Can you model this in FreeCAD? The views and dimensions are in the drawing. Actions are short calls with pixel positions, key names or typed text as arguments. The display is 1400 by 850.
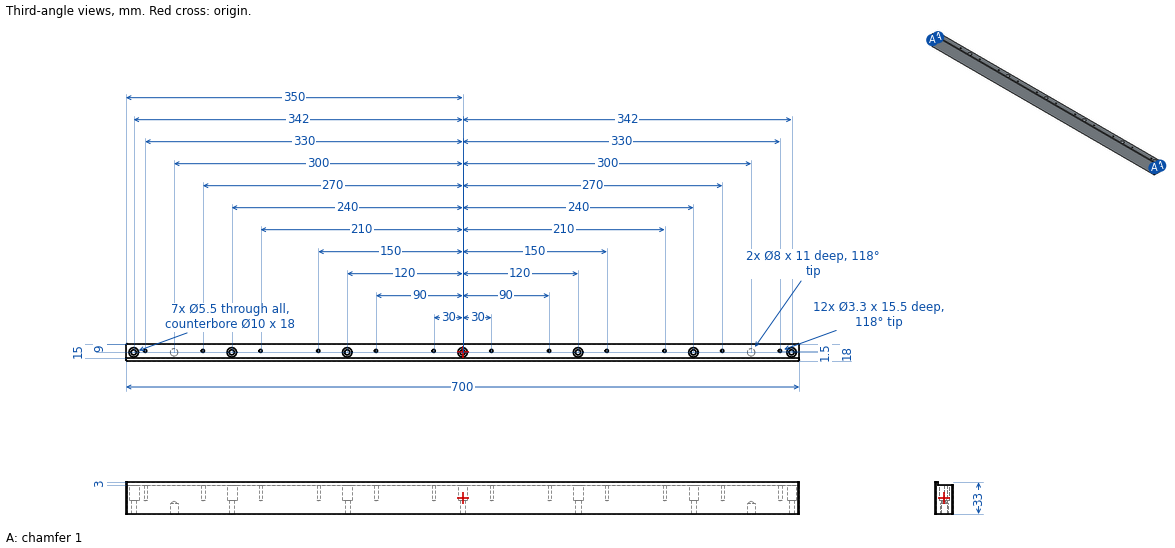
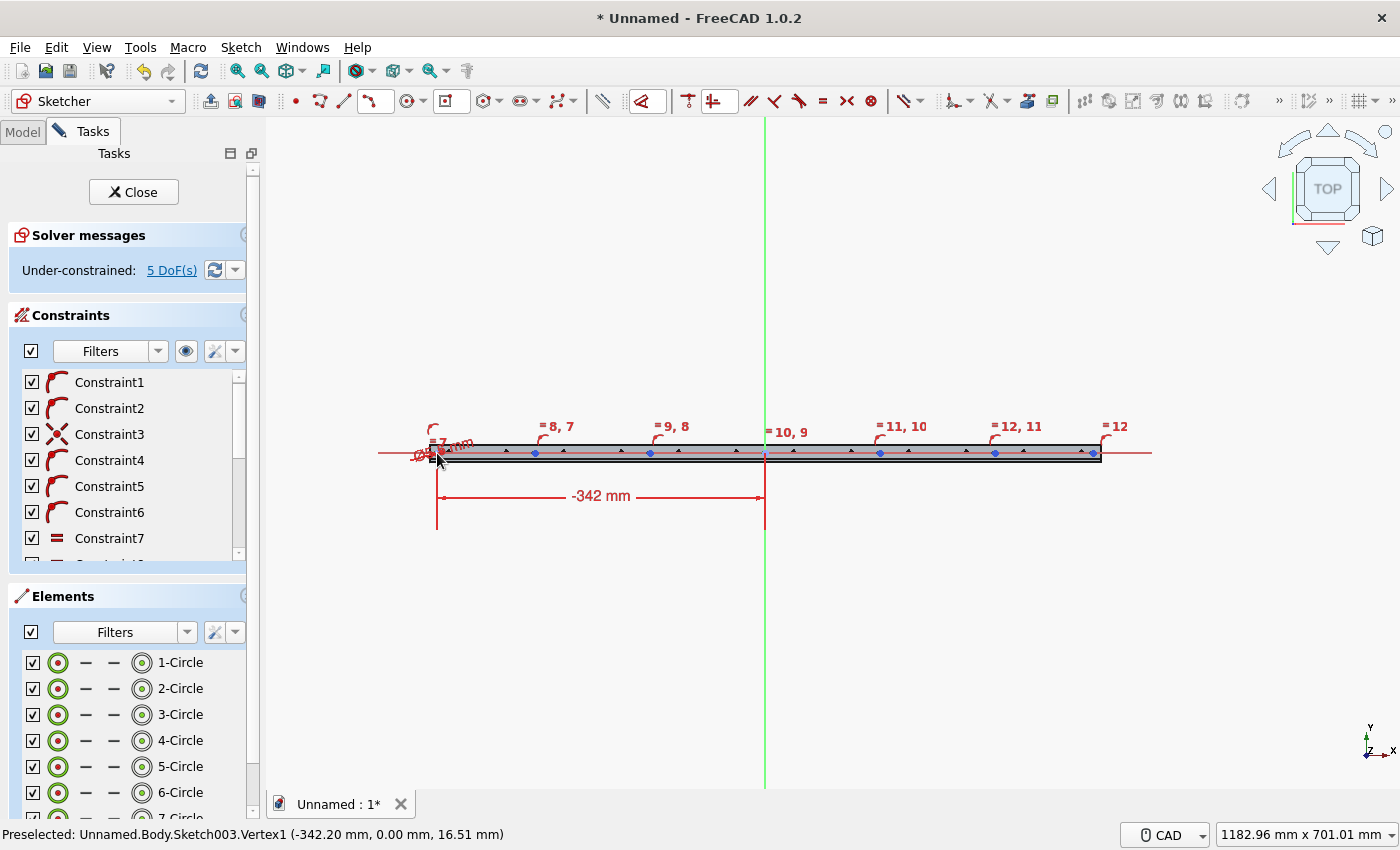
click(535, 453)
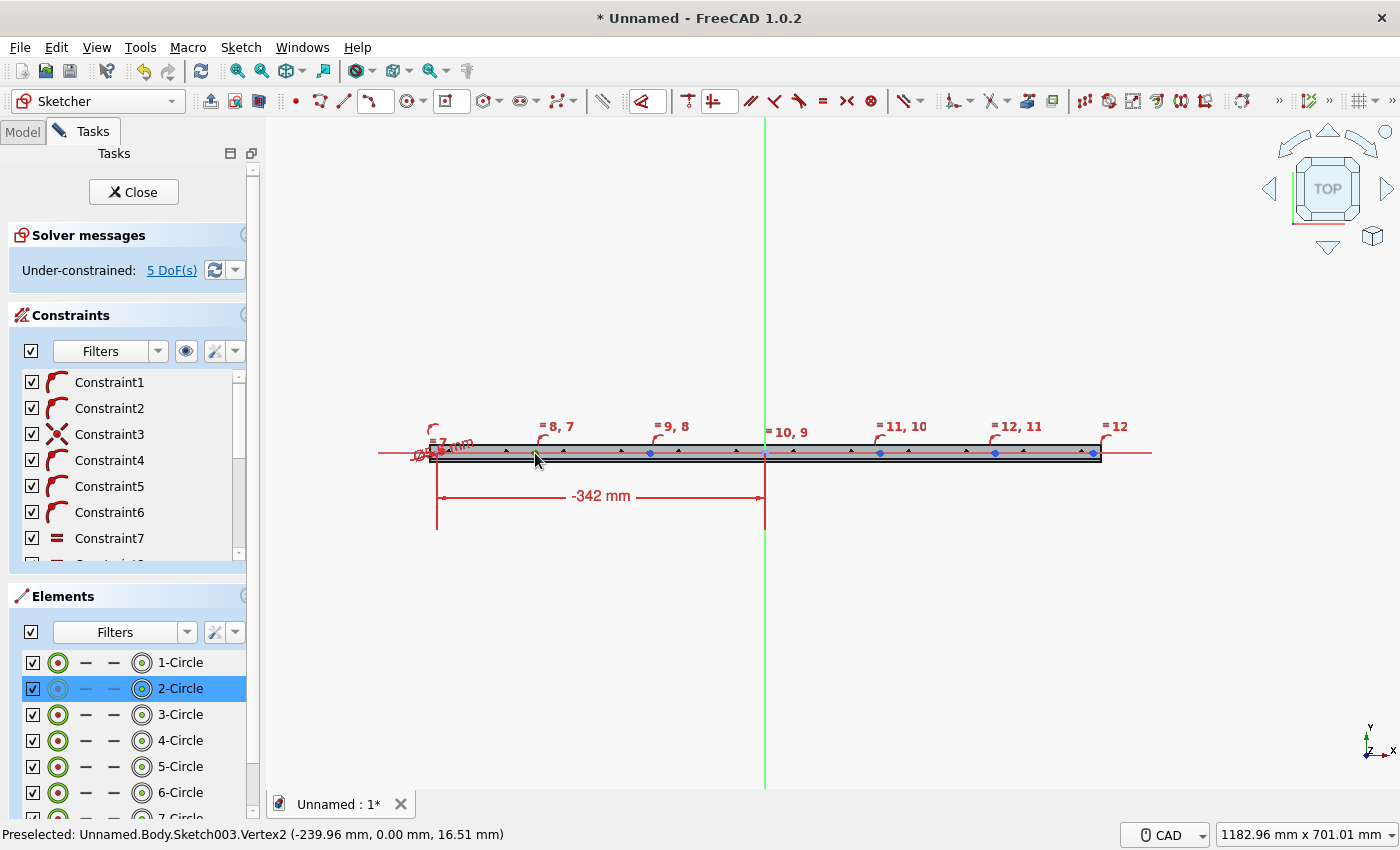
click(660, 102)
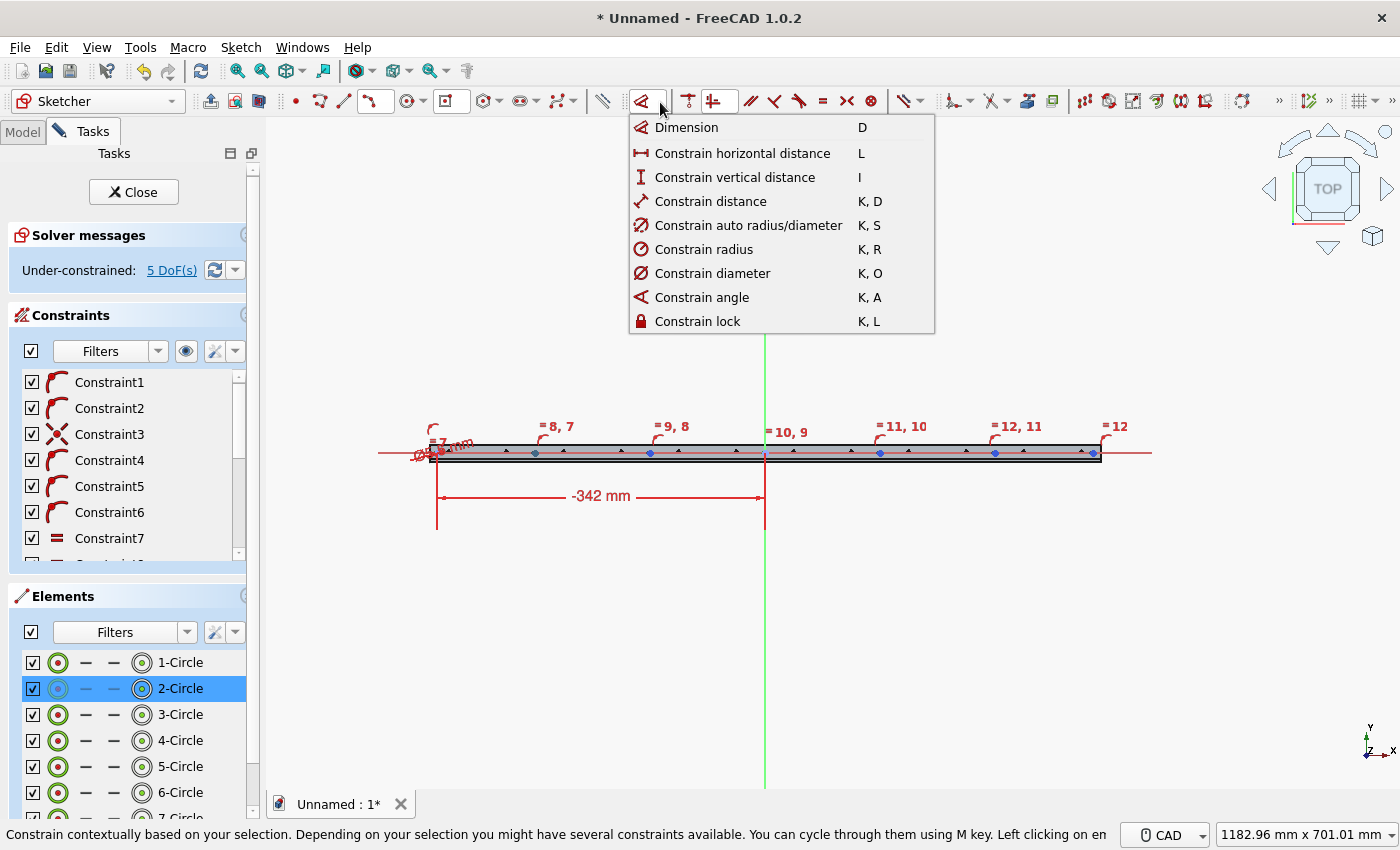
click(782, 153)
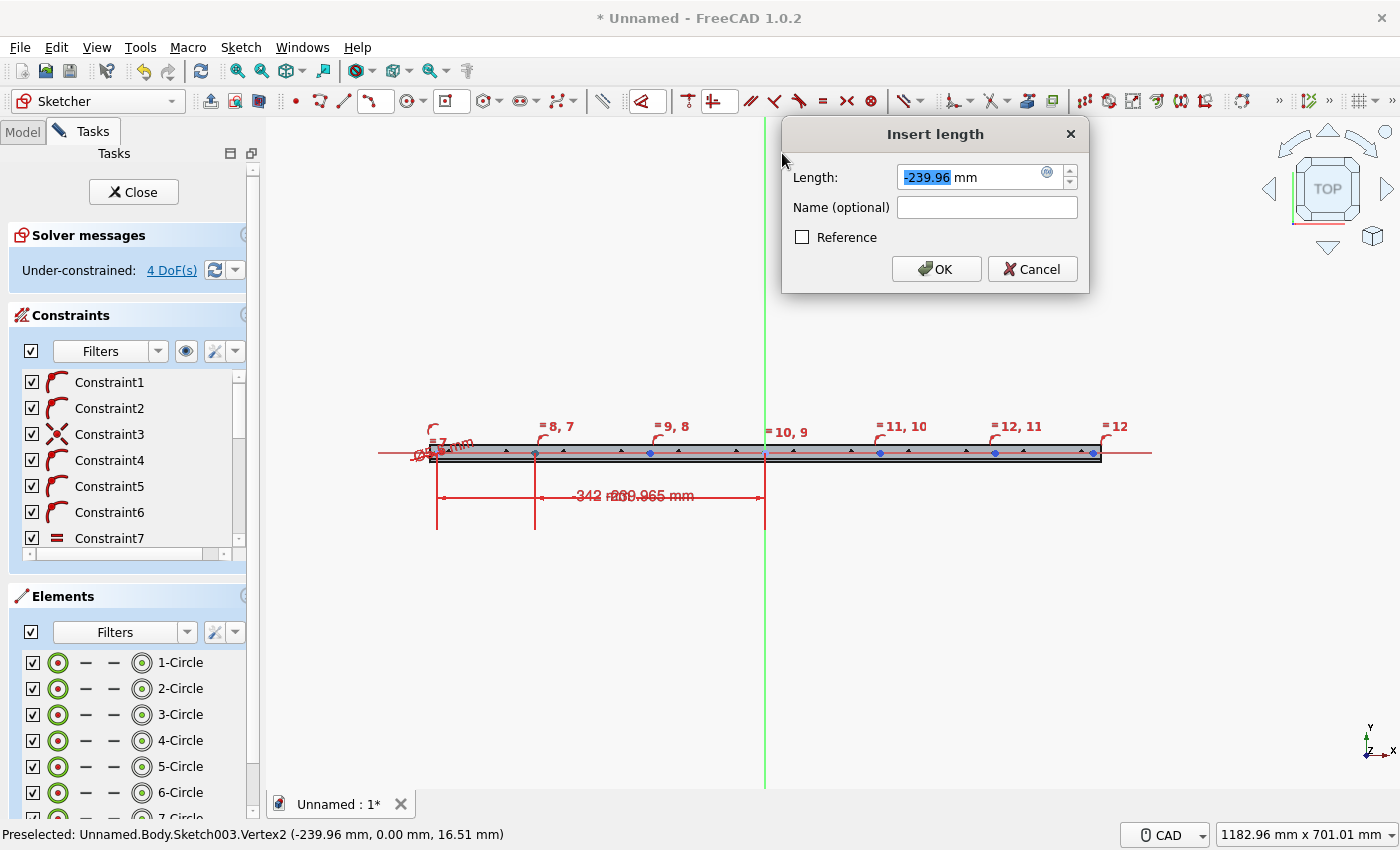
text(-240)
key(Return)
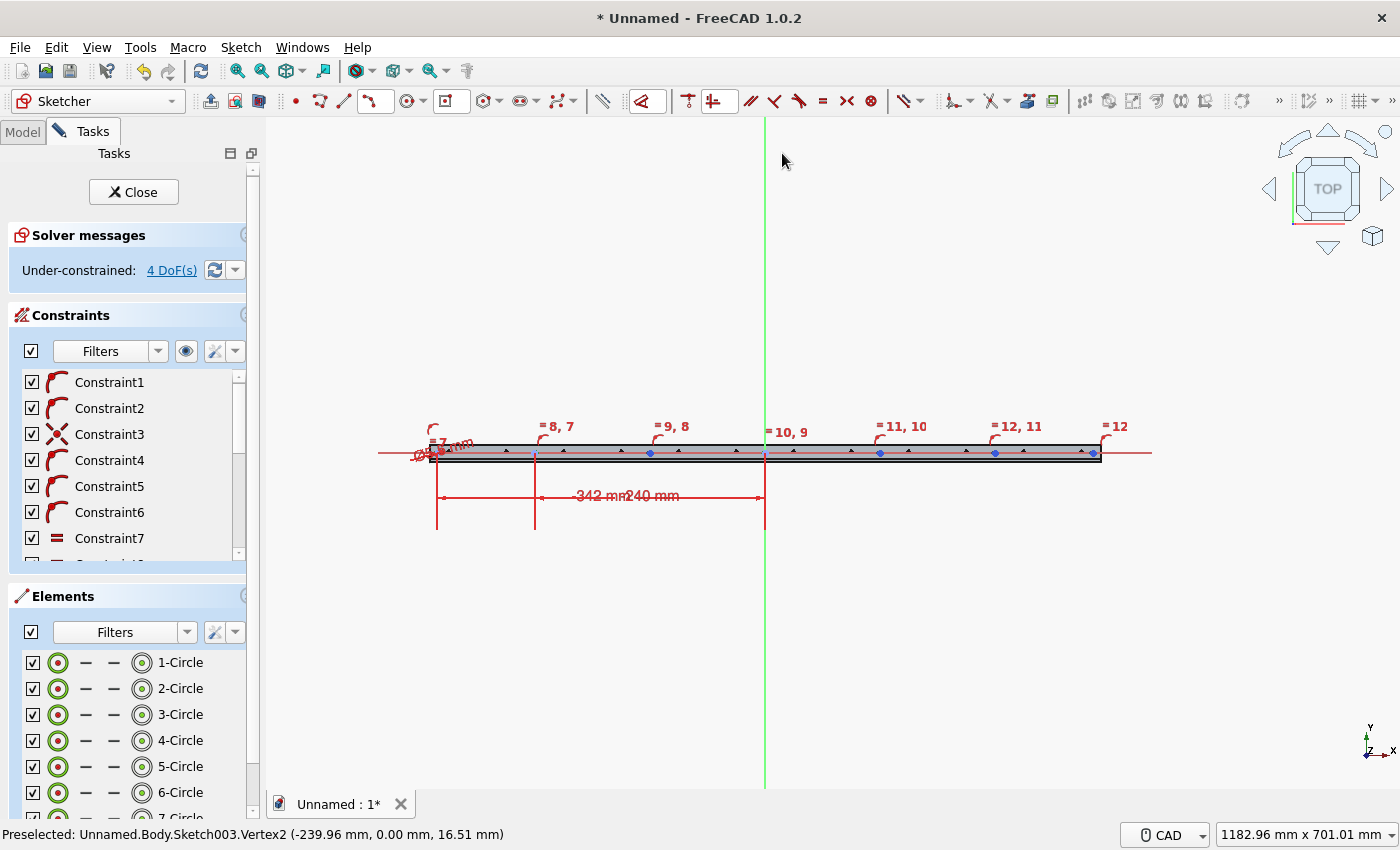
click(650, 453)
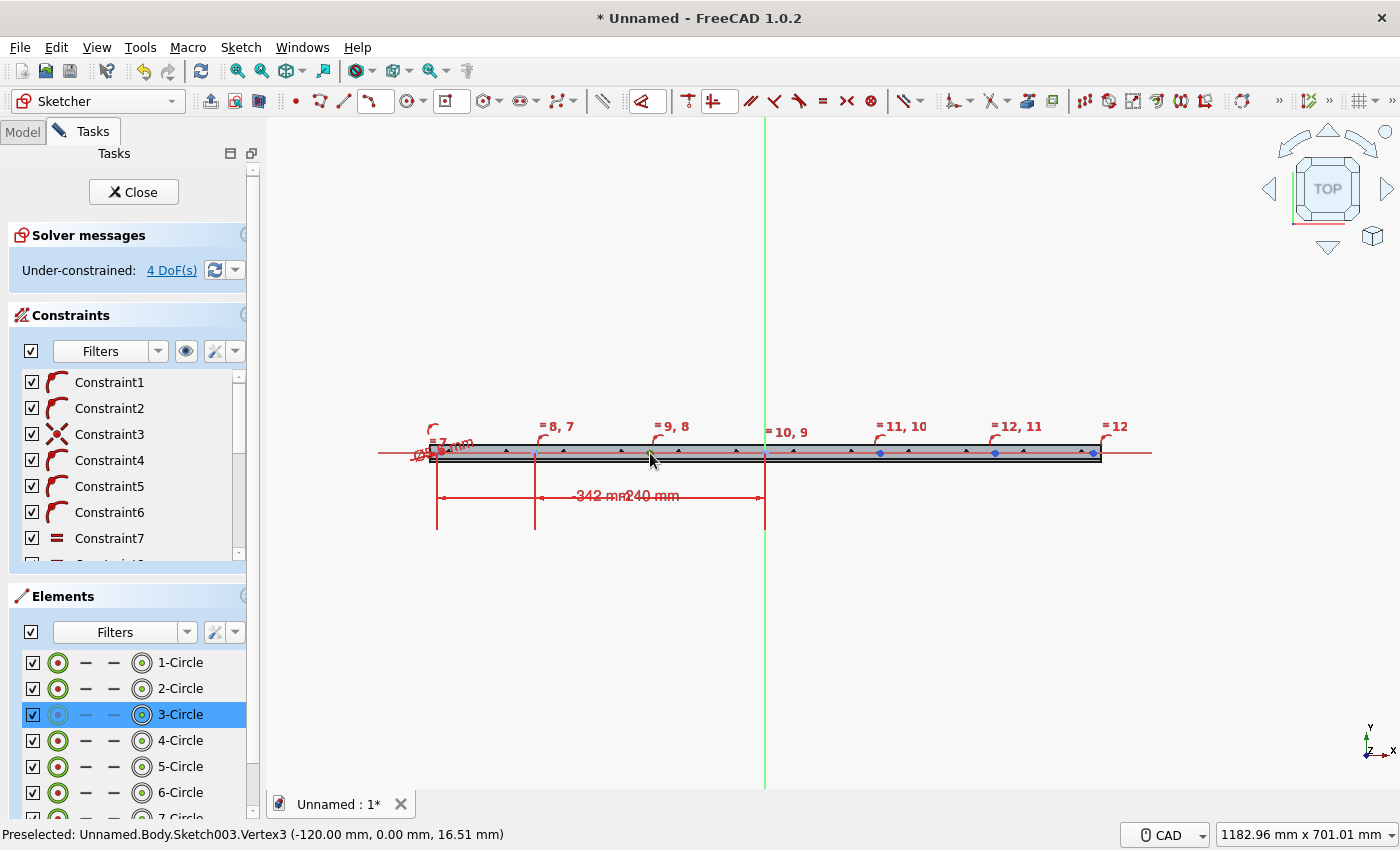
click(660, 102)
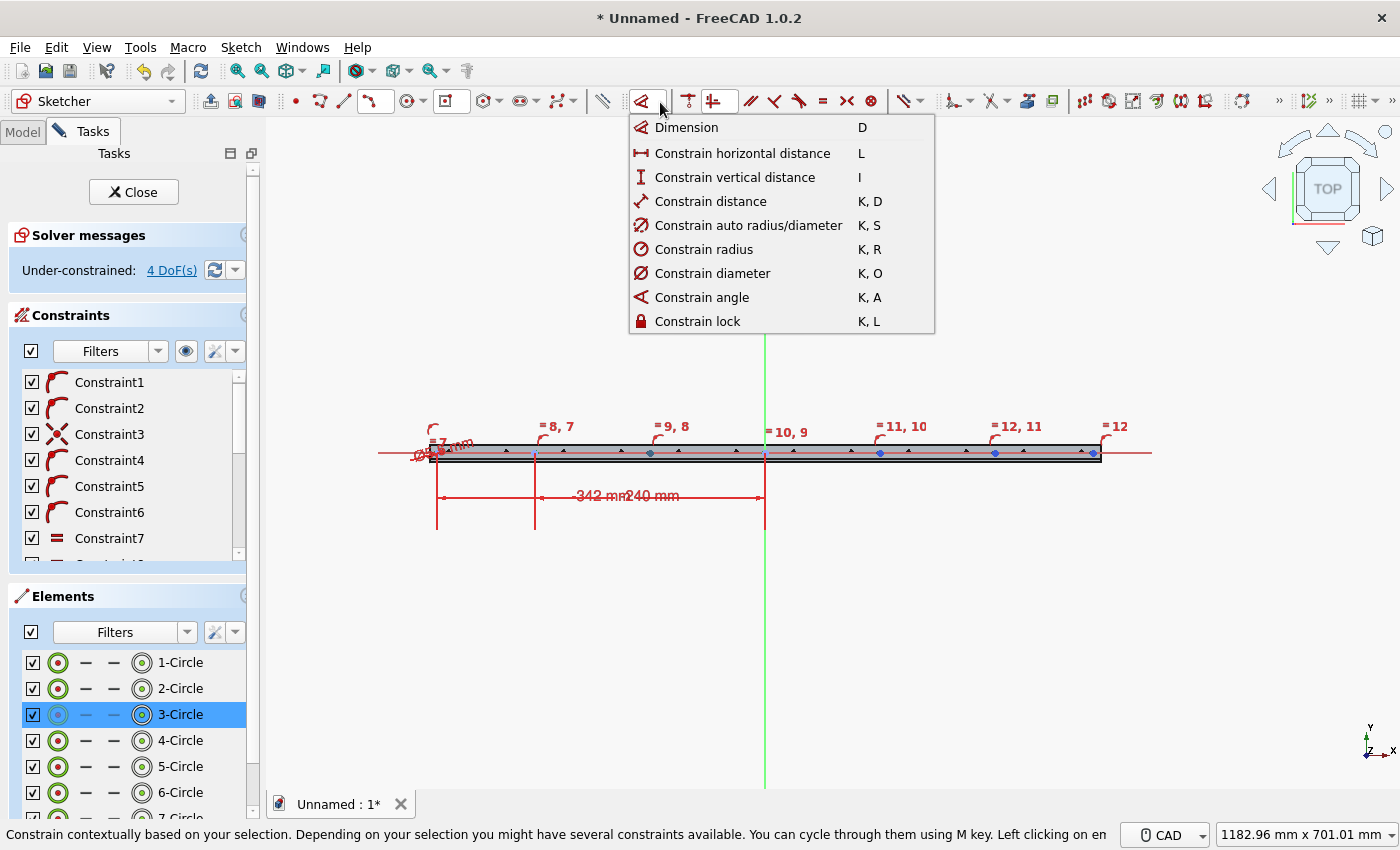
click(782, 153)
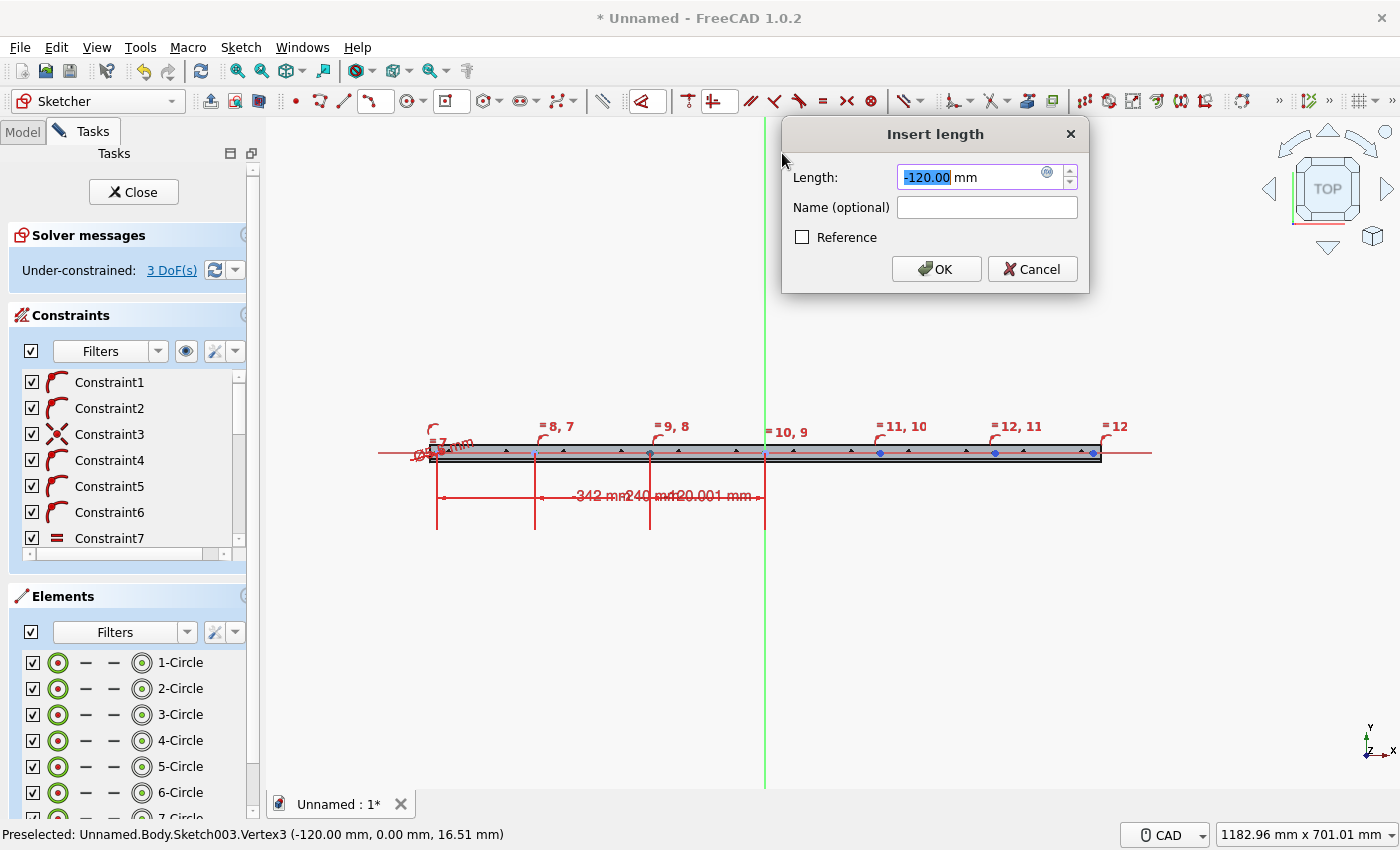
text(-120)
key(Return)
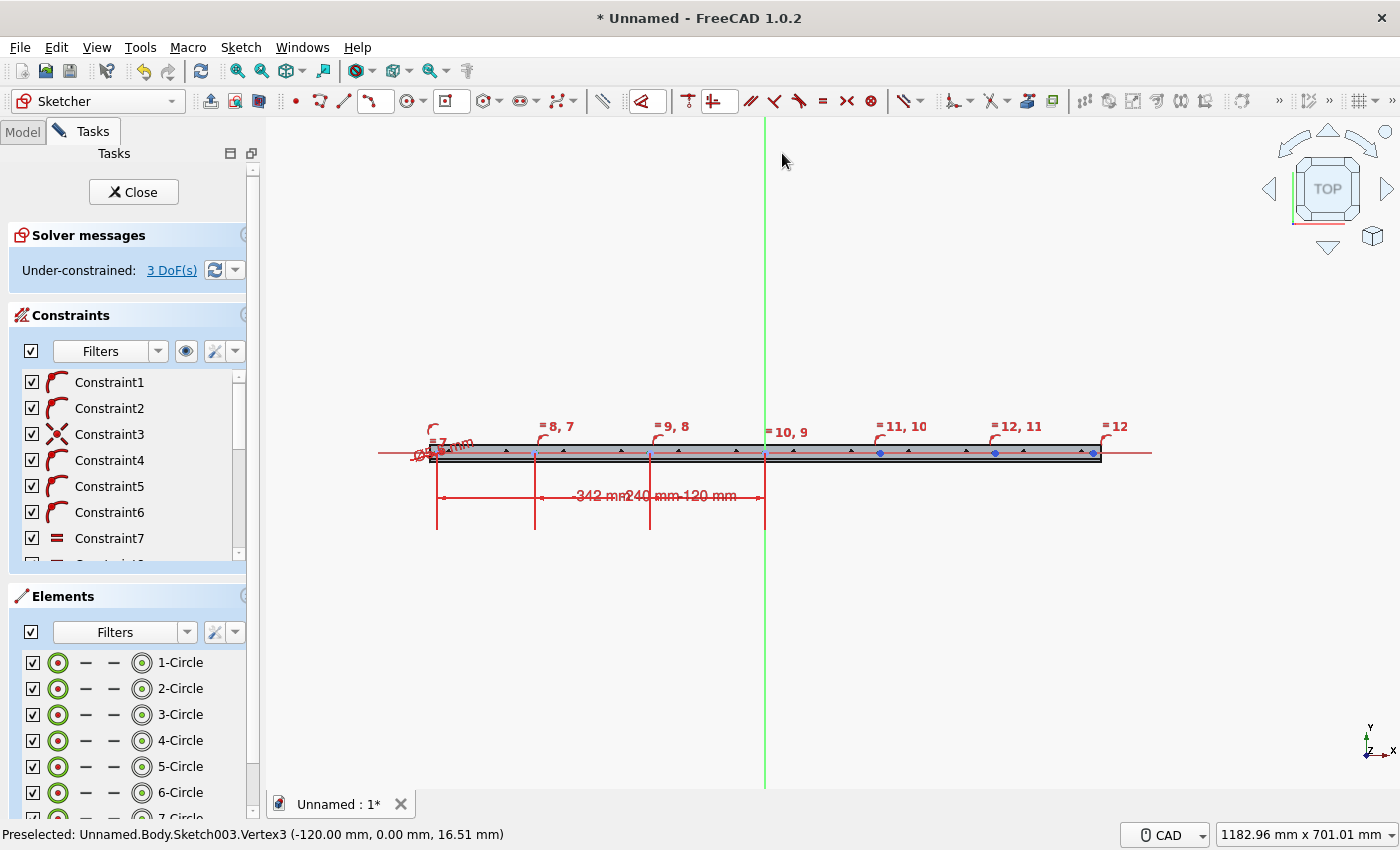
click(880, 453)